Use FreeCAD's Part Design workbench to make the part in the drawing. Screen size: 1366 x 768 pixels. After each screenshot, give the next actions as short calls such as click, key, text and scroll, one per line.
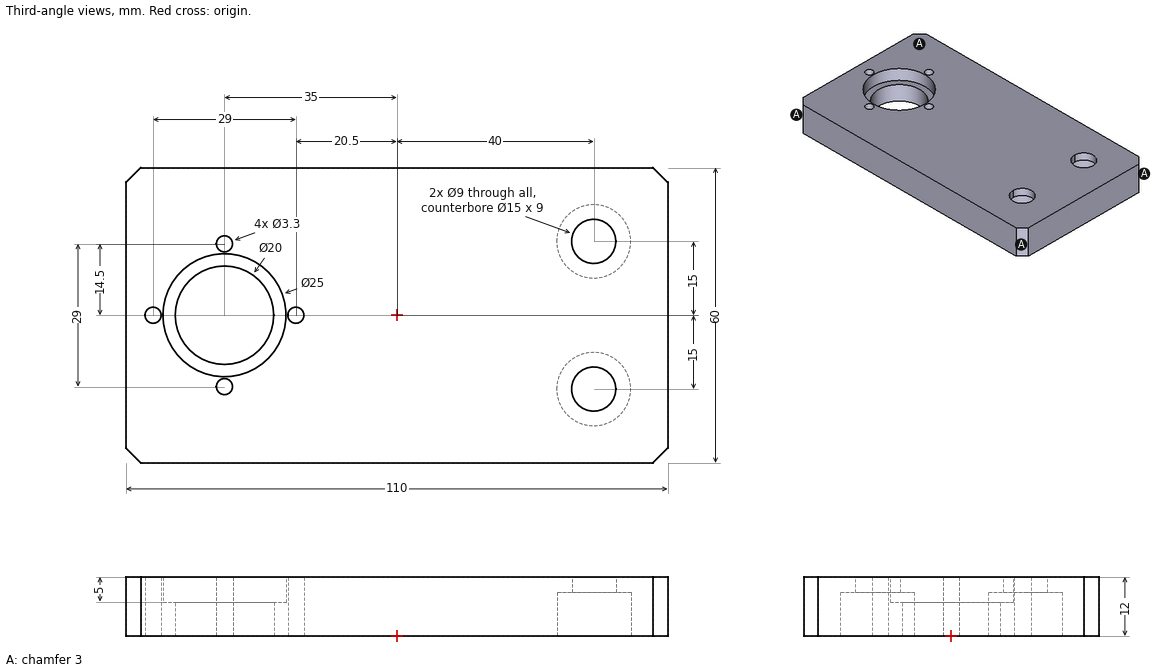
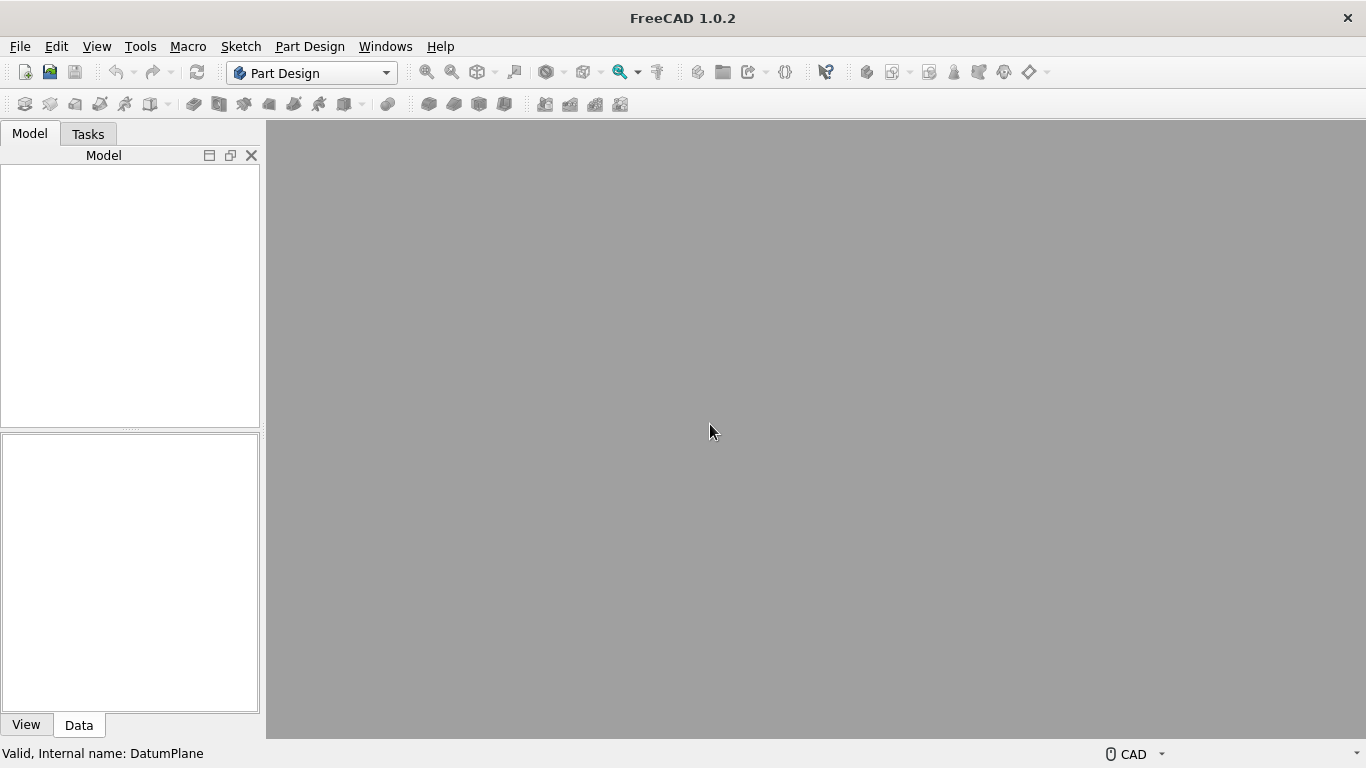
key(ctrl+n)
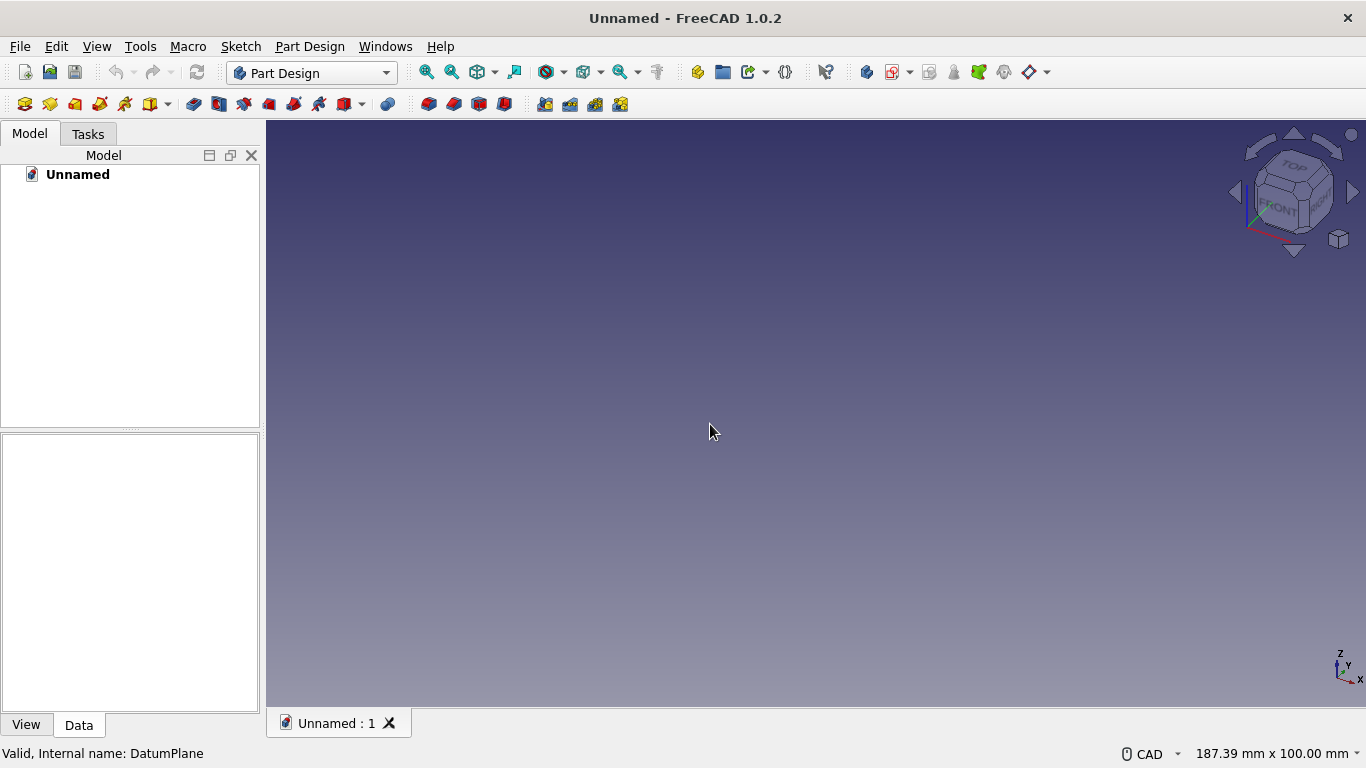
click(892, 72)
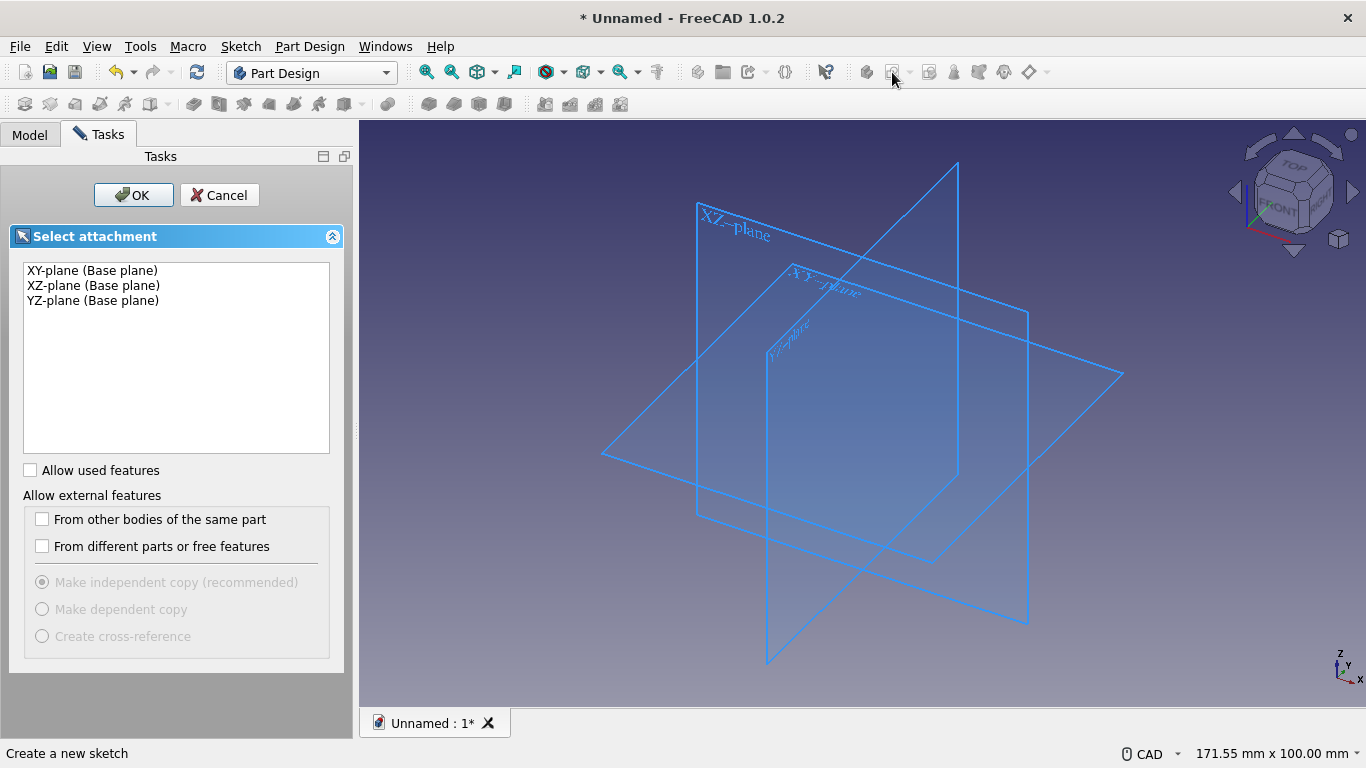
click(84, 270)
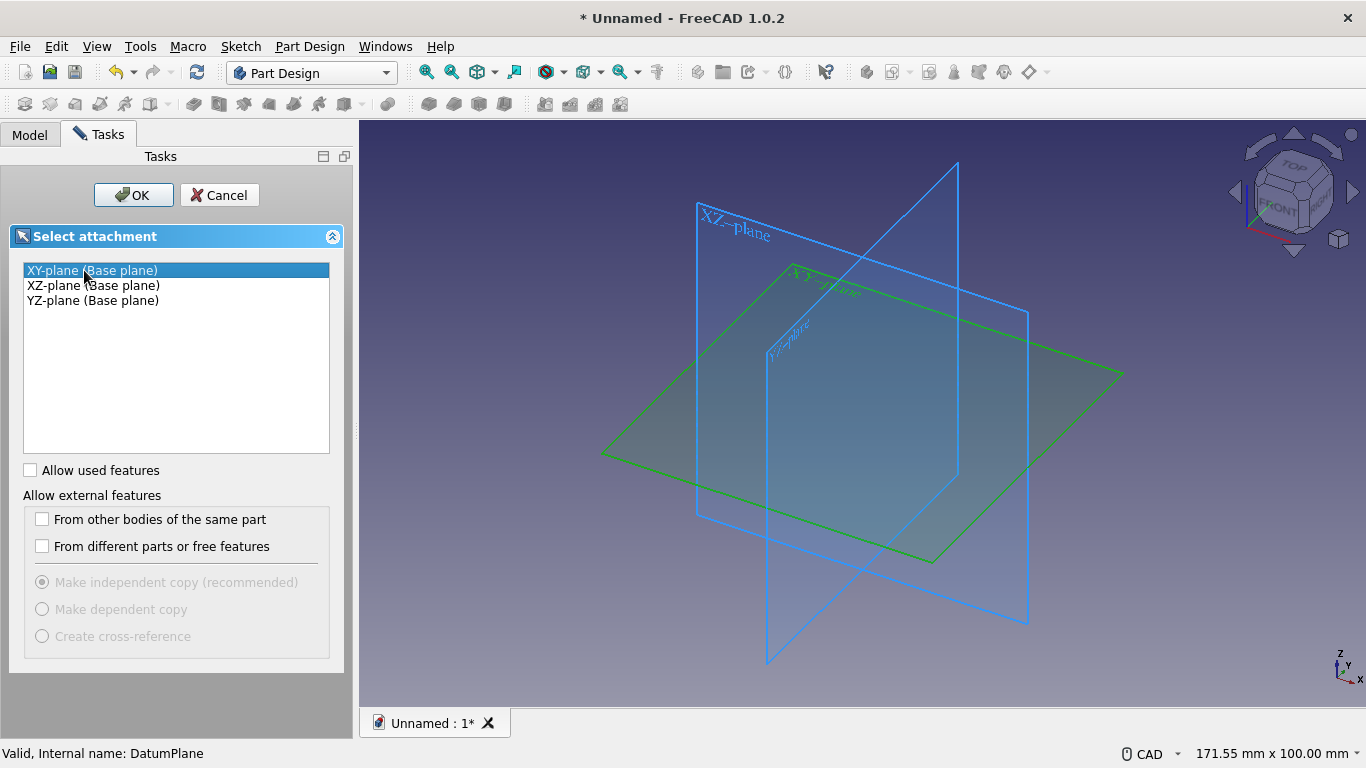
click(134, 195)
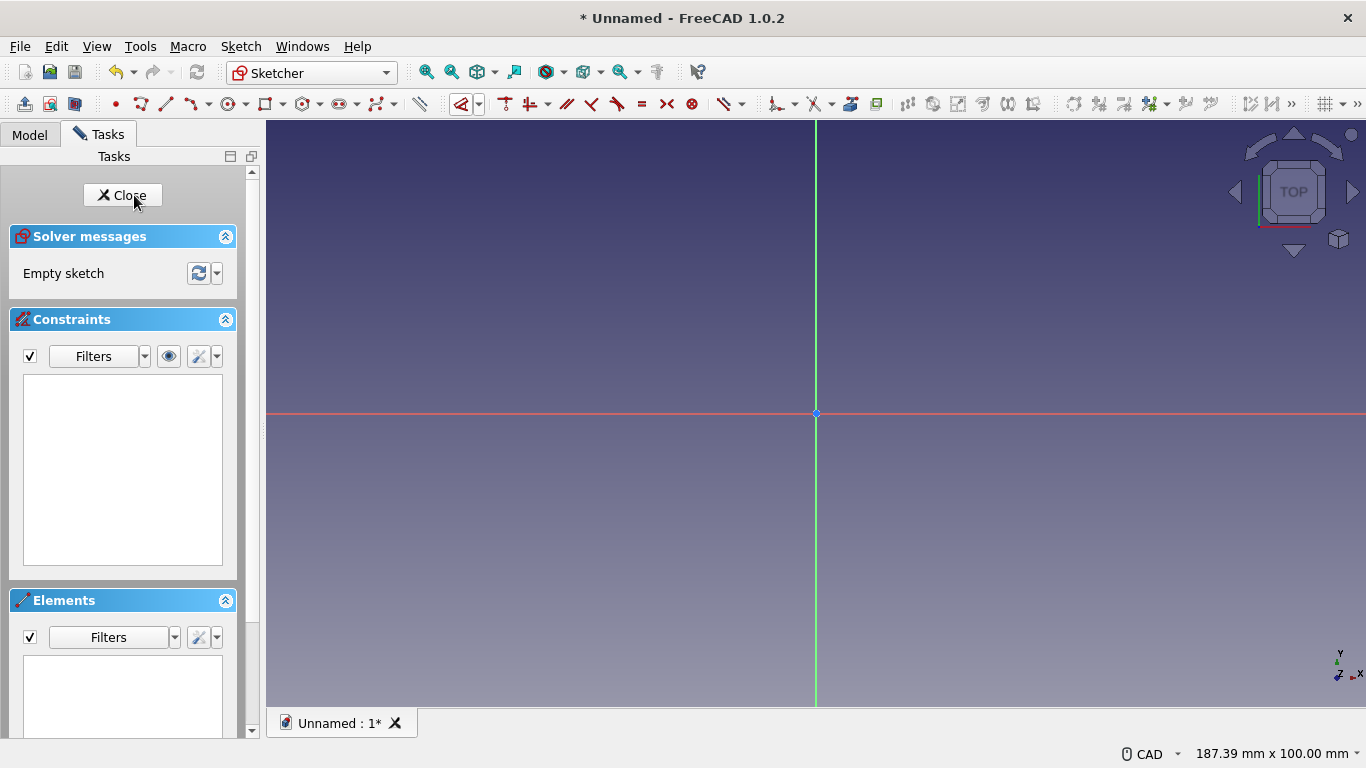
click(282, 104)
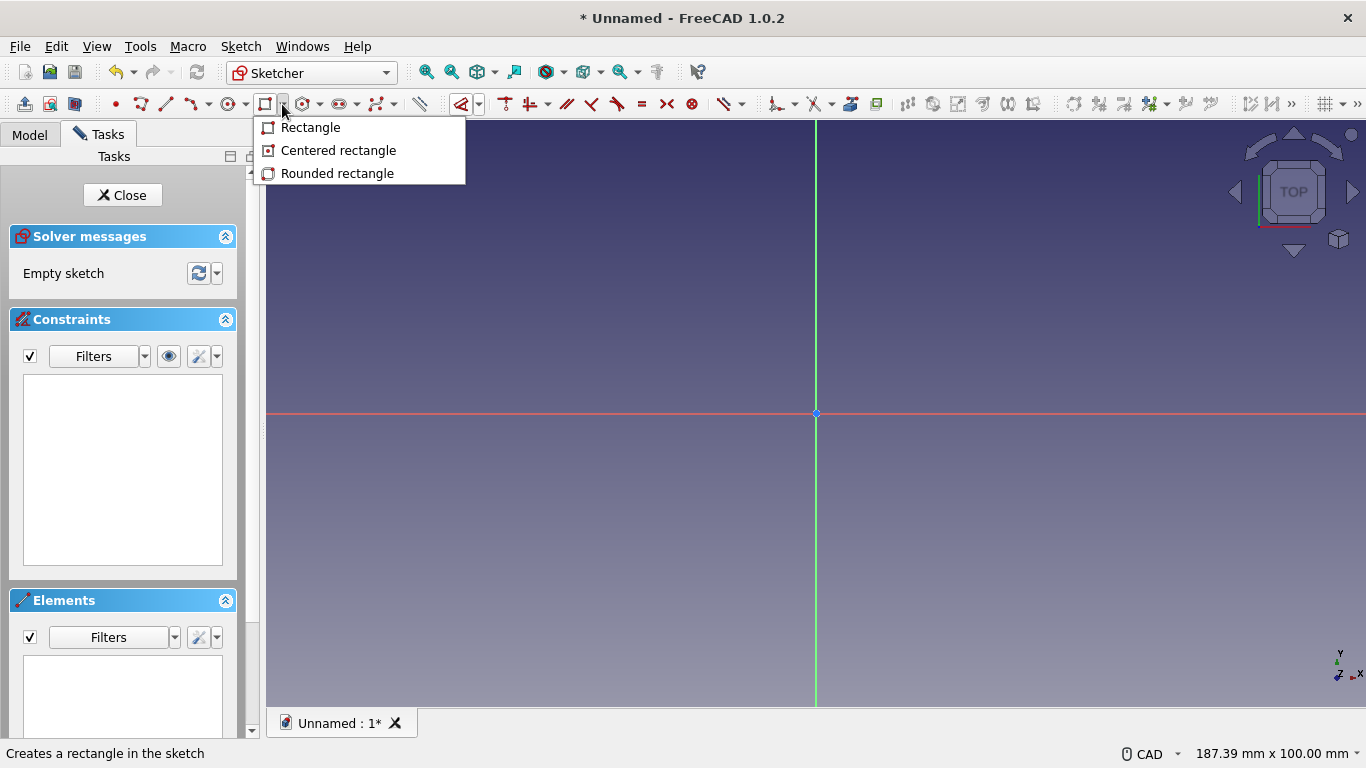
click(360, 150)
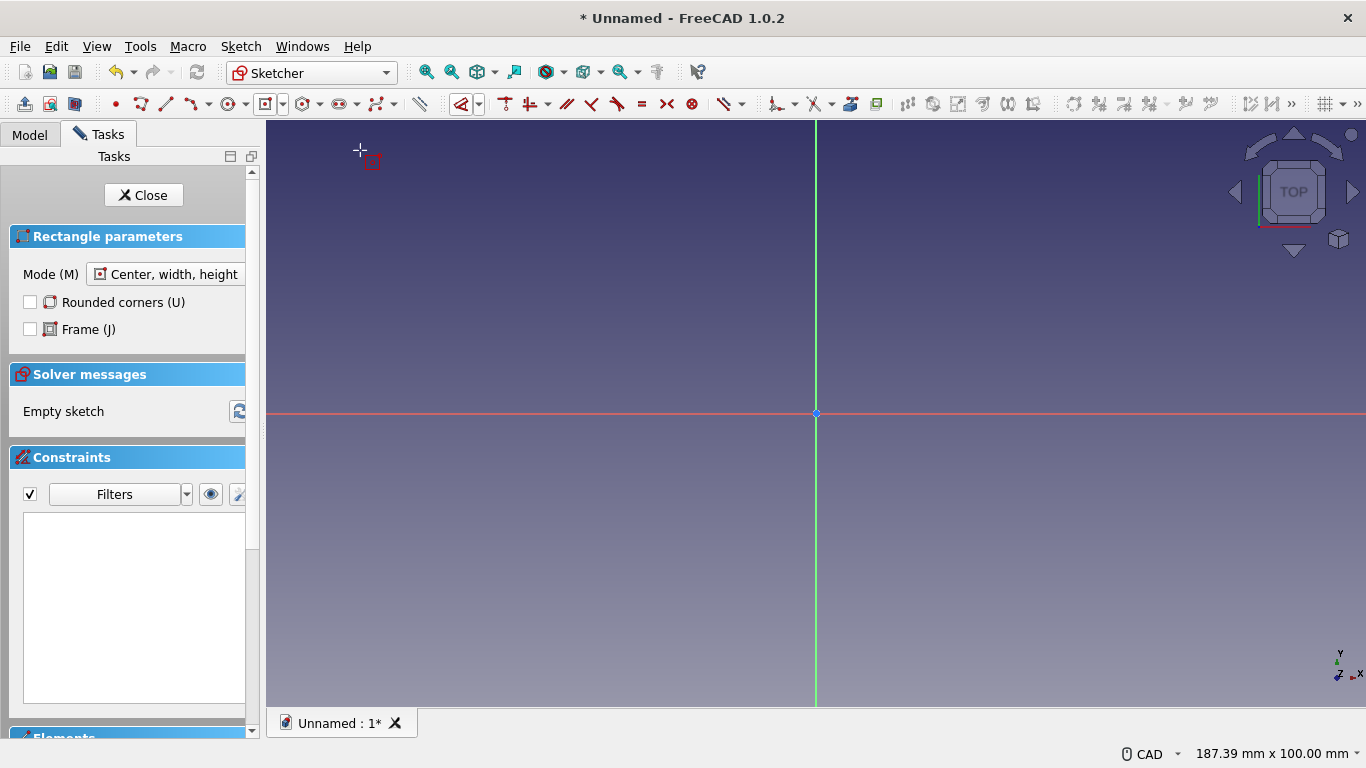
click(816, 414)
click(1139, 237)
key(Escape)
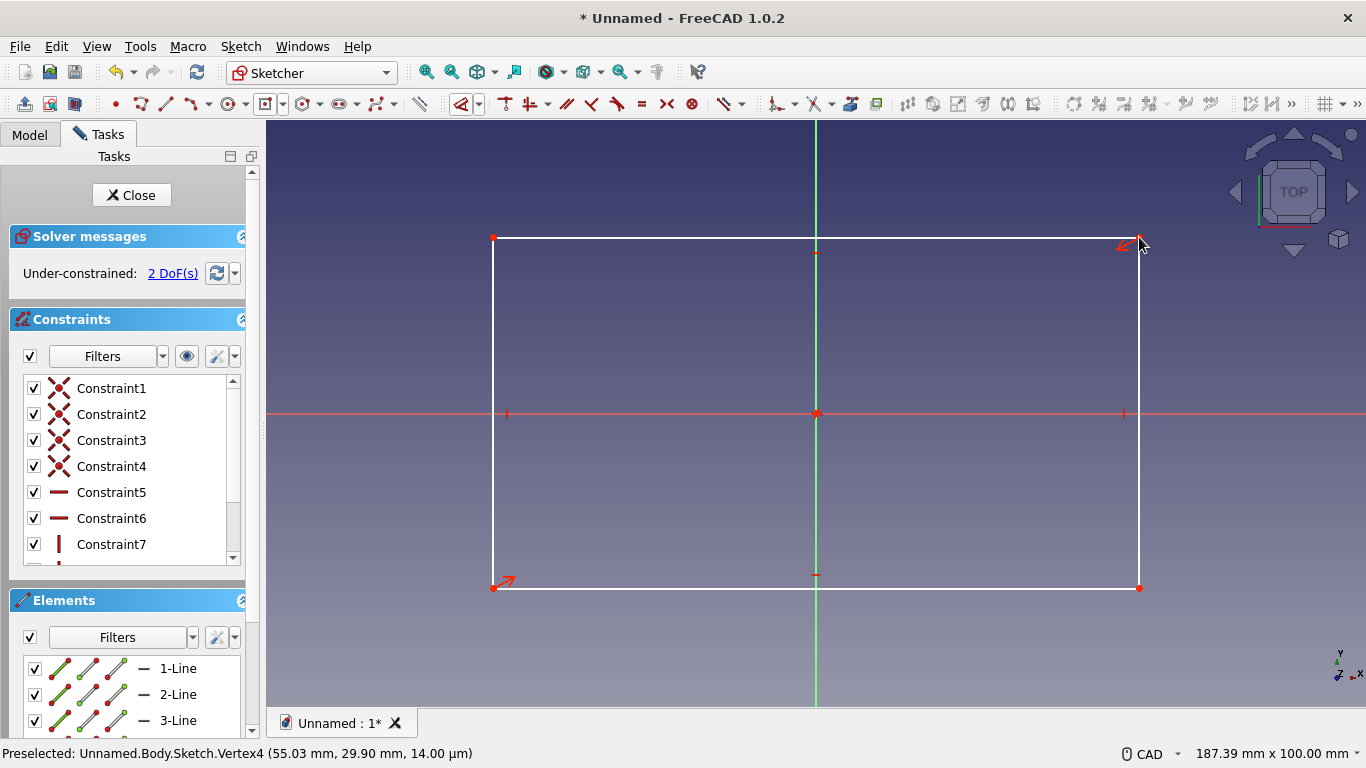
key(d)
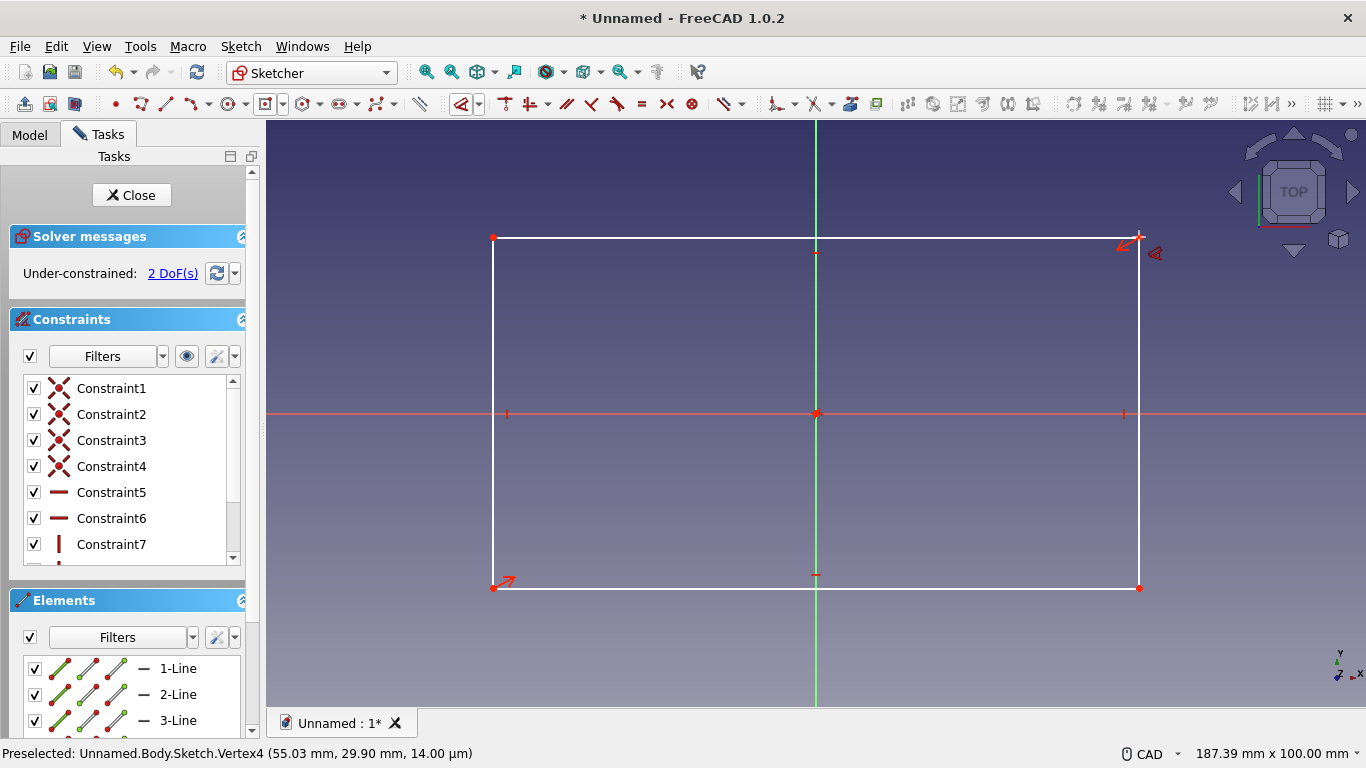
click(1139, 484)
click(1173, 333)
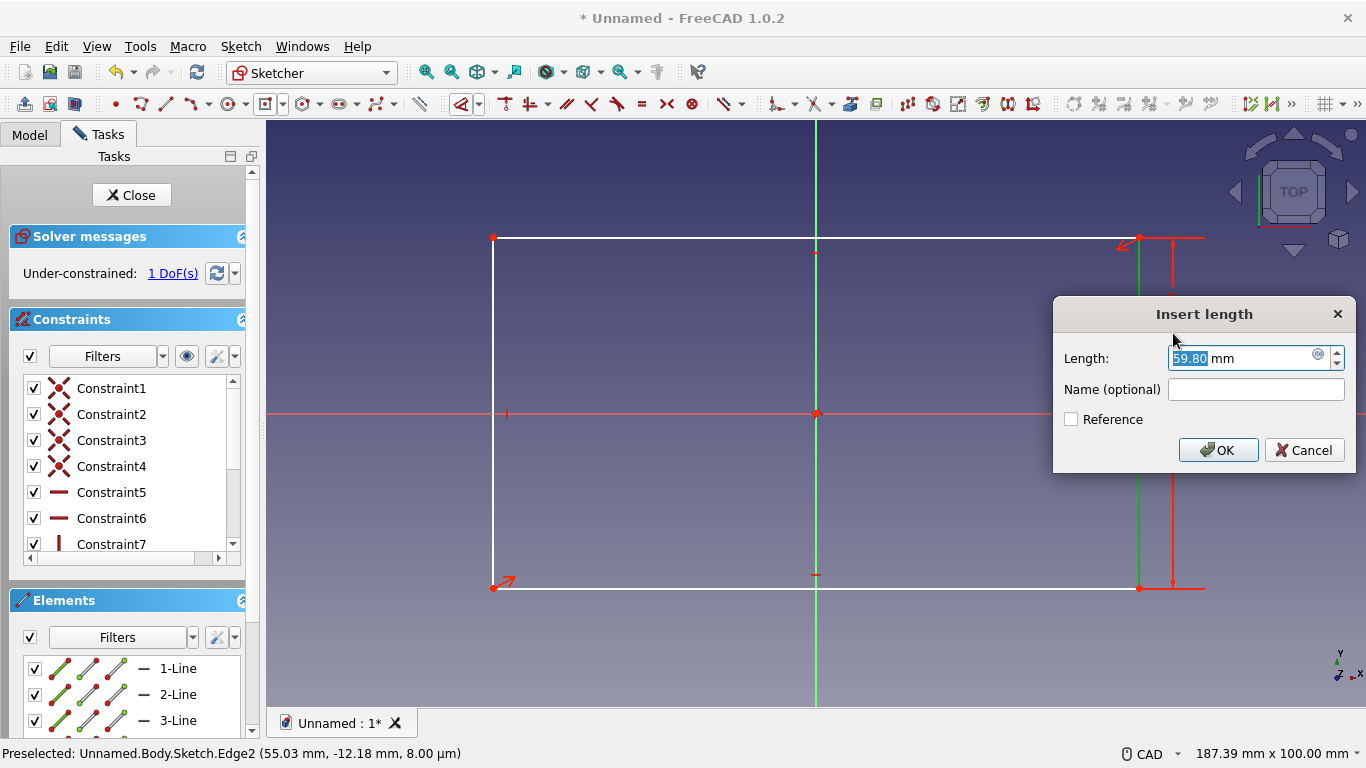
text(60)
key(Return)